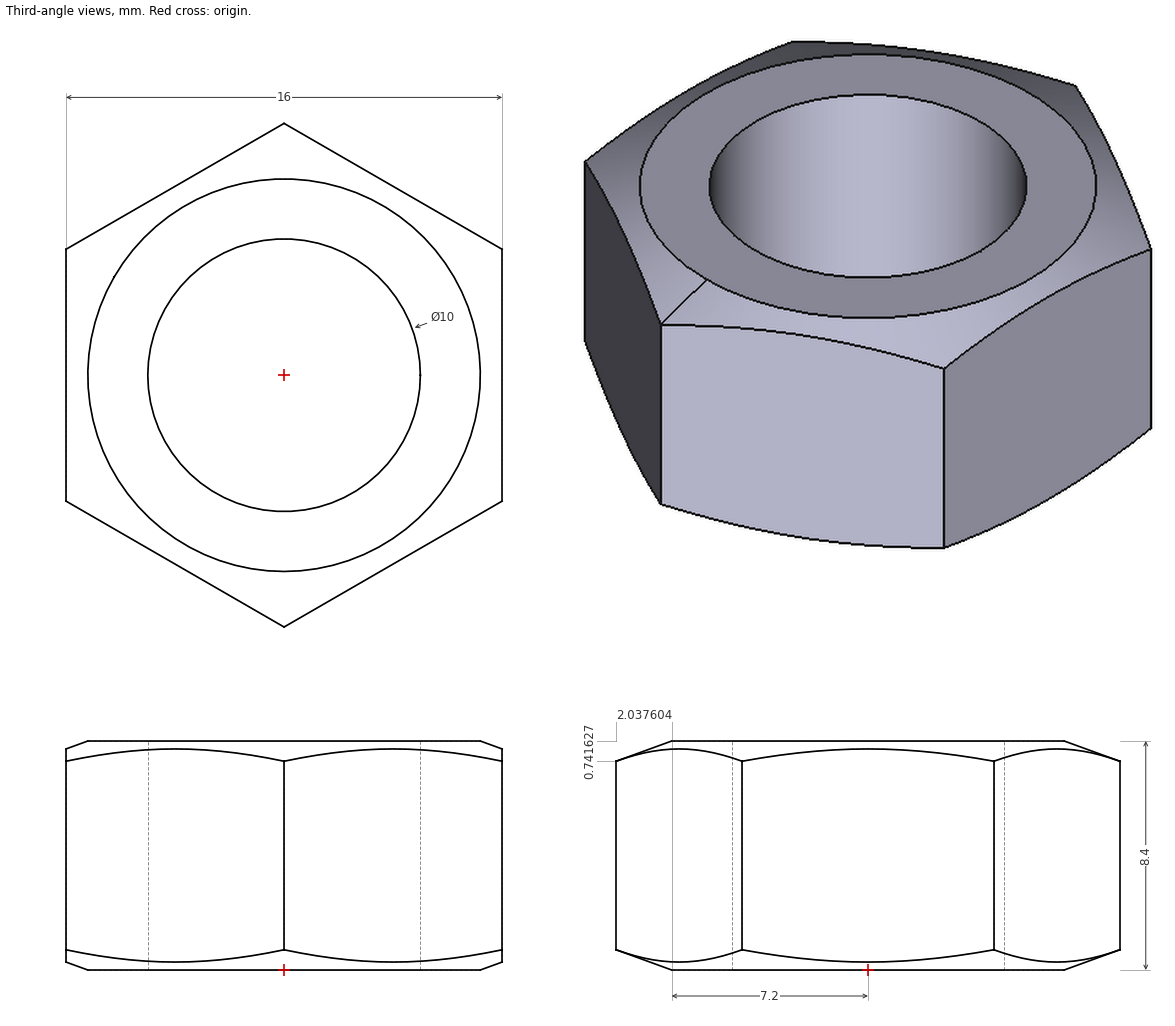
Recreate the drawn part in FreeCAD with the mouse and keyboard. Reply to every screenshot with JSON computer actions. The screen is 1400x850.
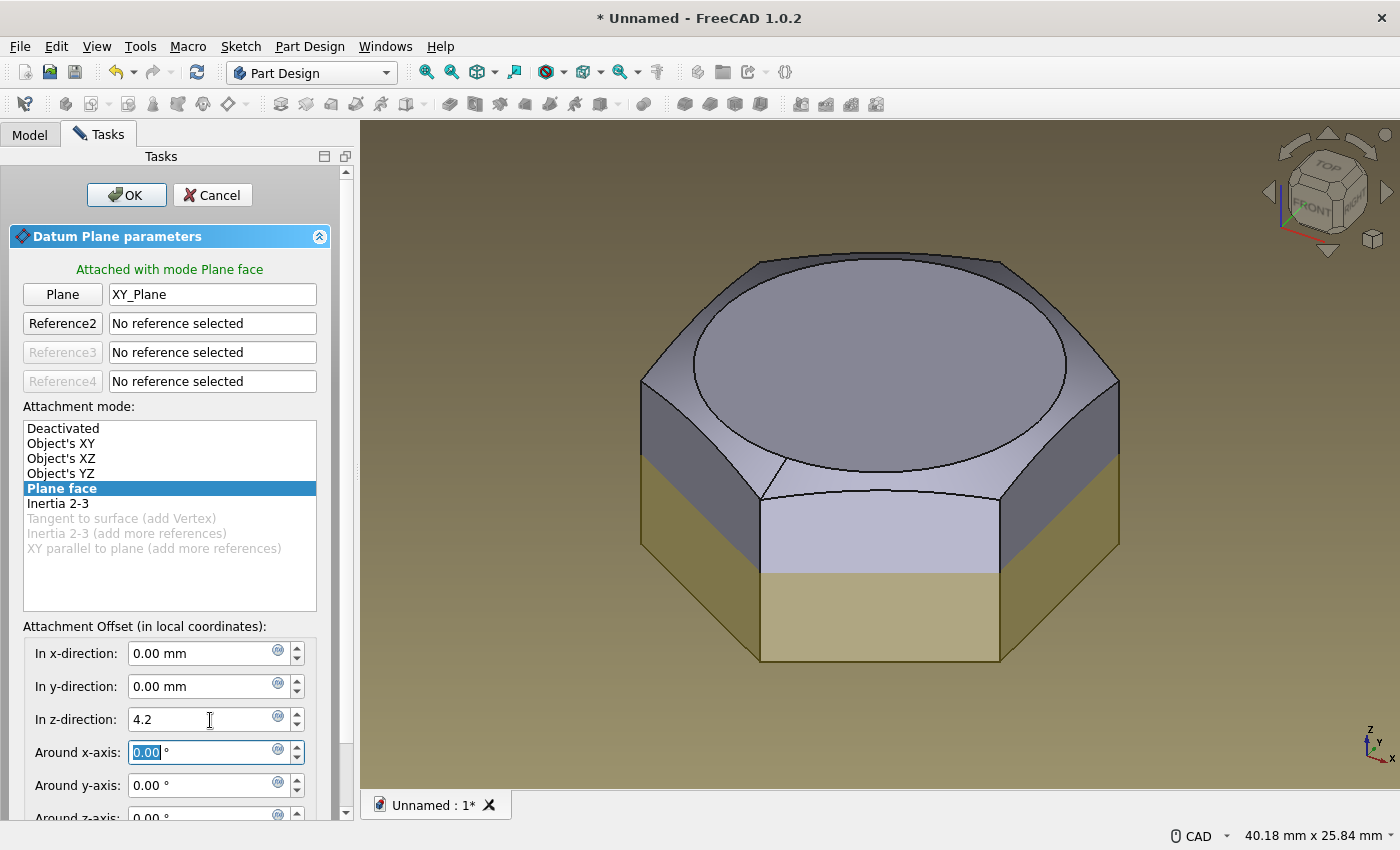
{"action": "left_click", "coordinate": [127, 195]}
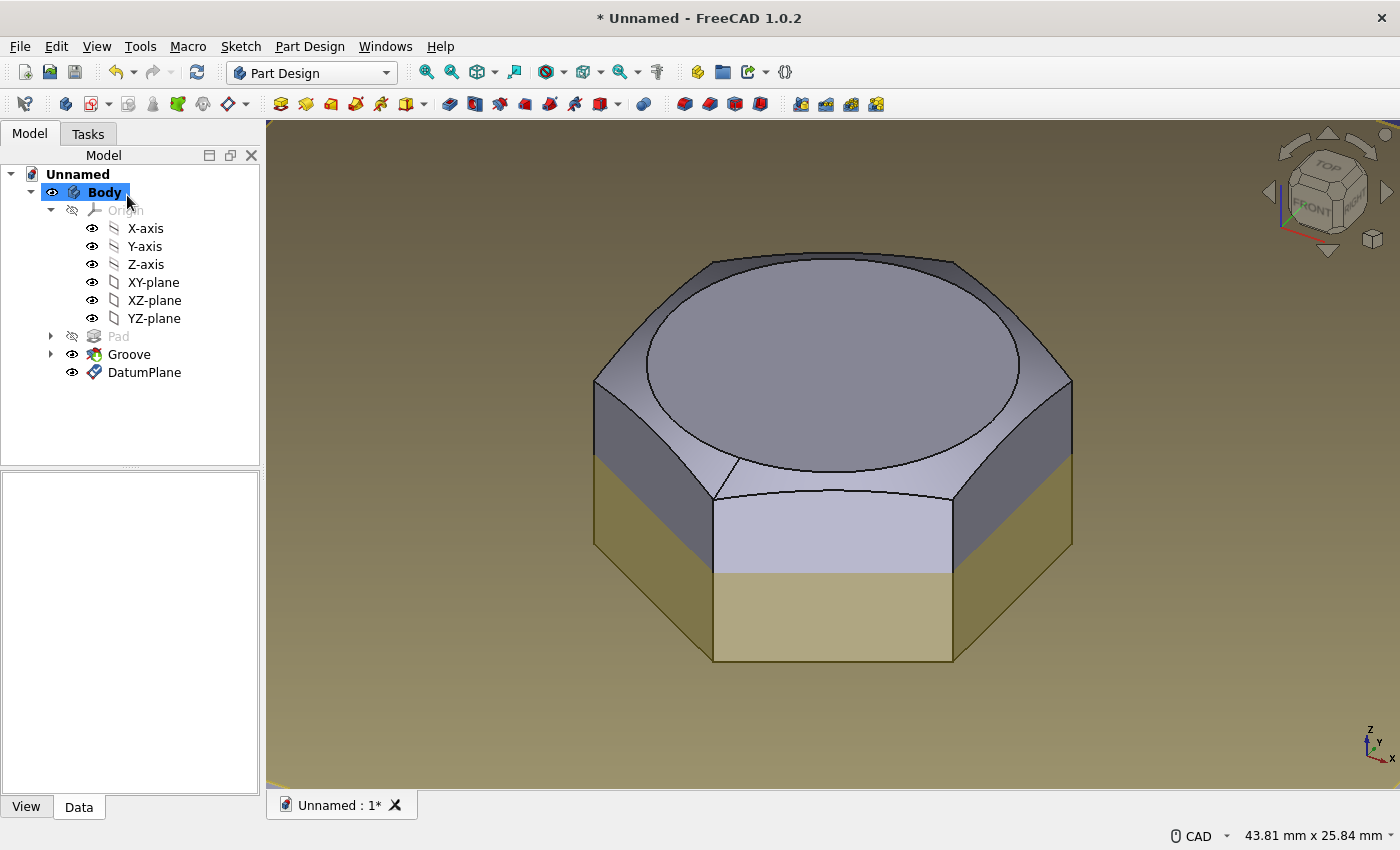
{"action": "left_click", "coordinate": [117, 354]}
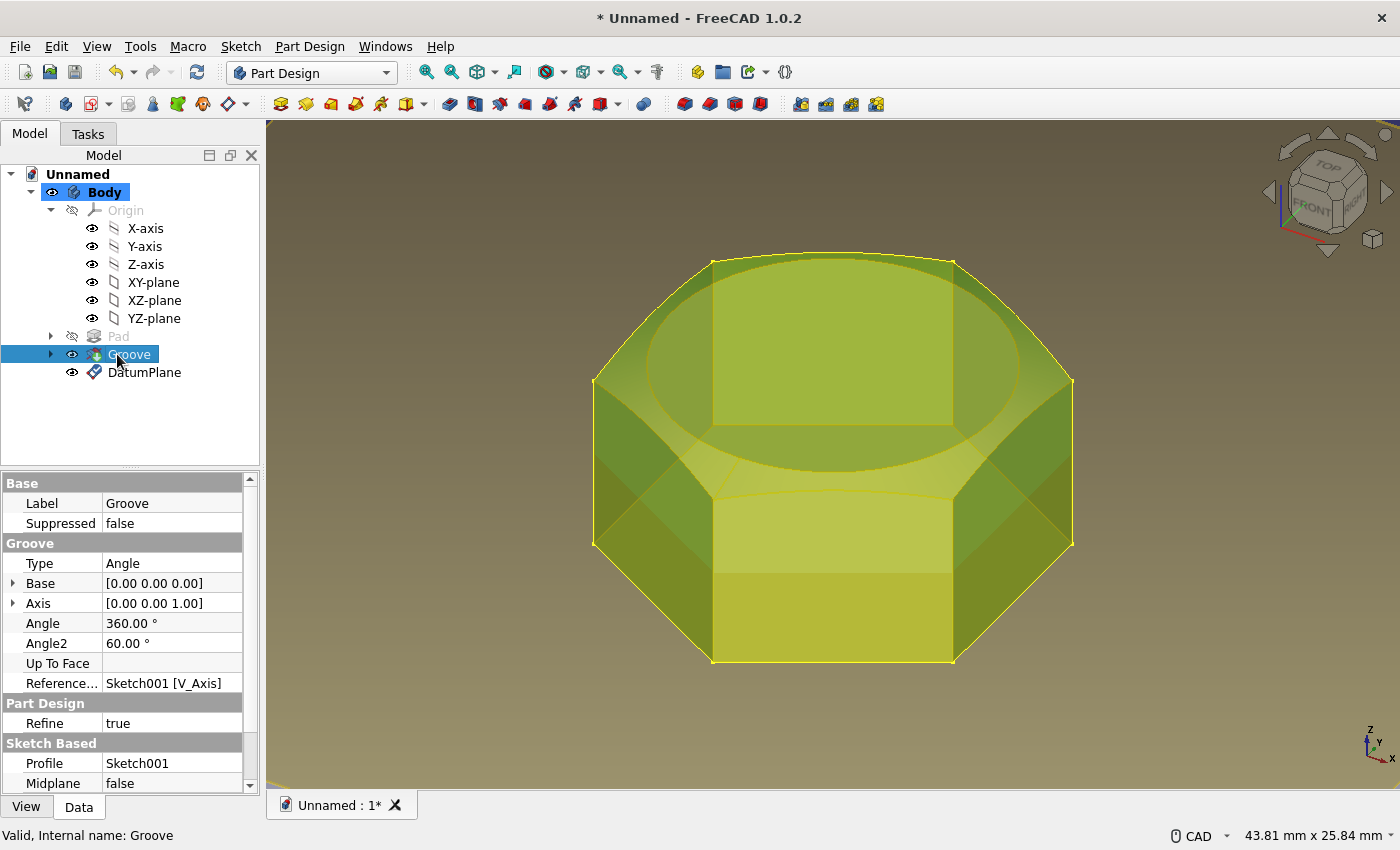
{"action": "left_click", "coordinate": [801, 104]}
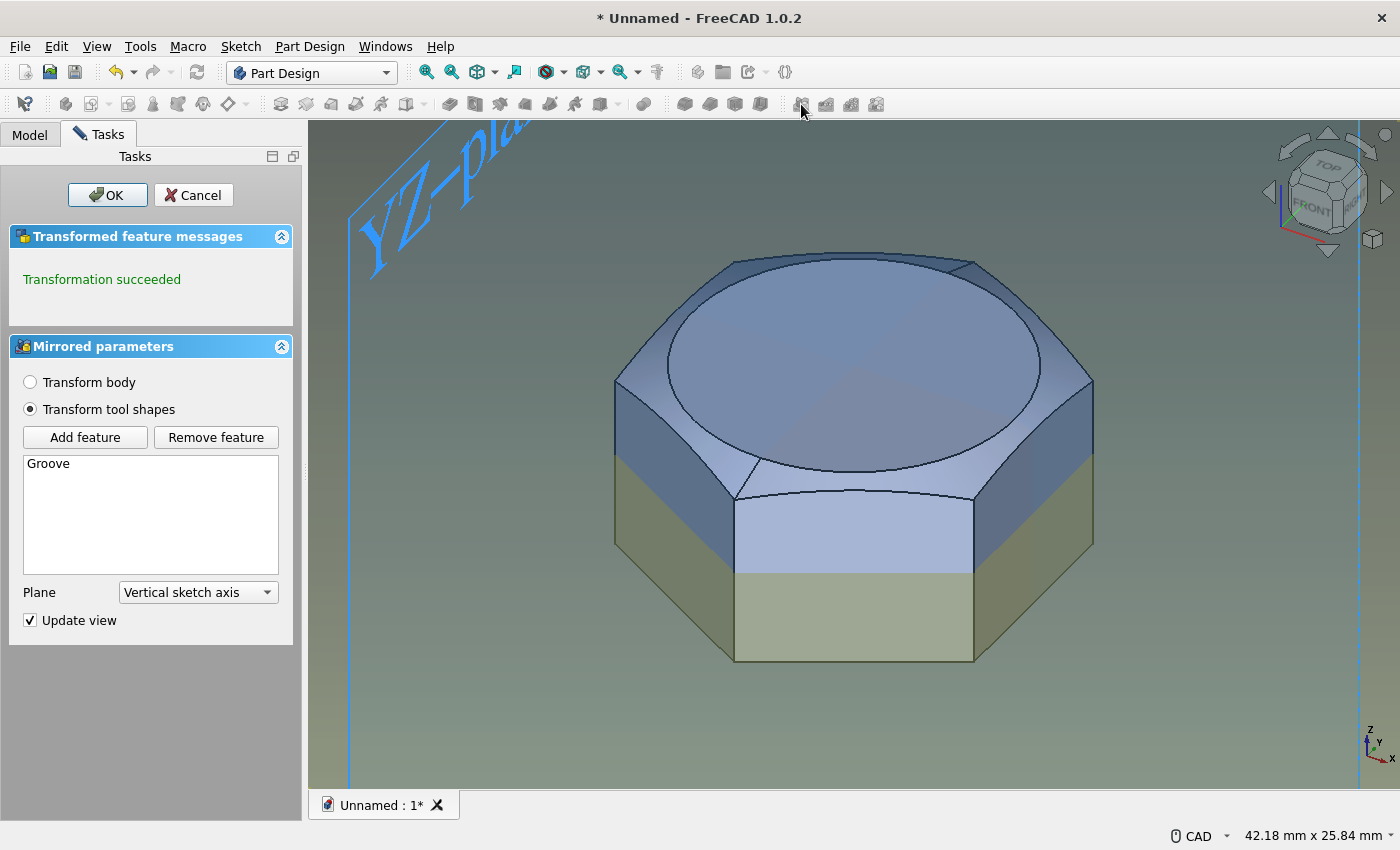
{"action": "left_click", "coordinate": [199, 592]}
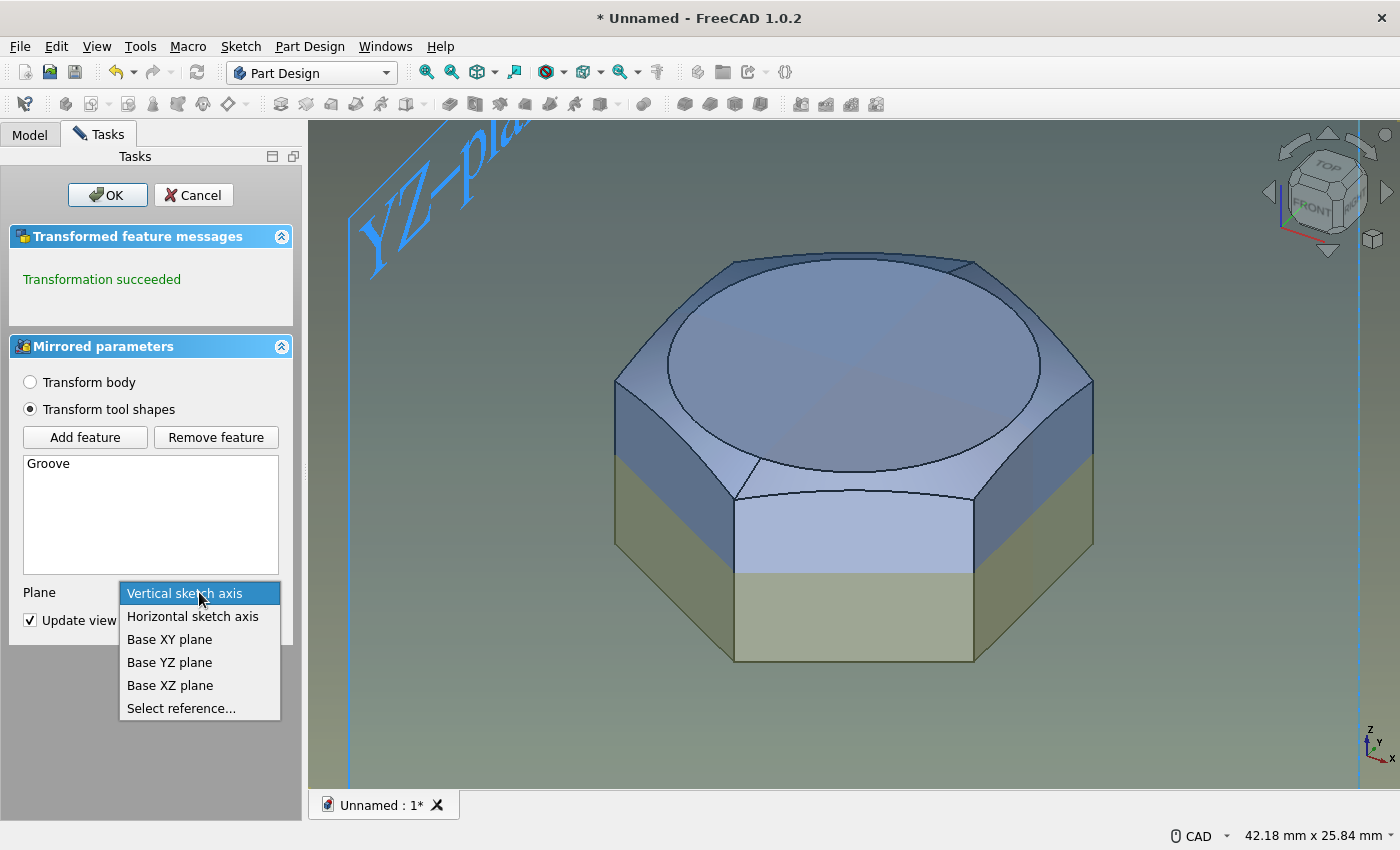
{"action": "left_click", "coordinate": [198, 708]}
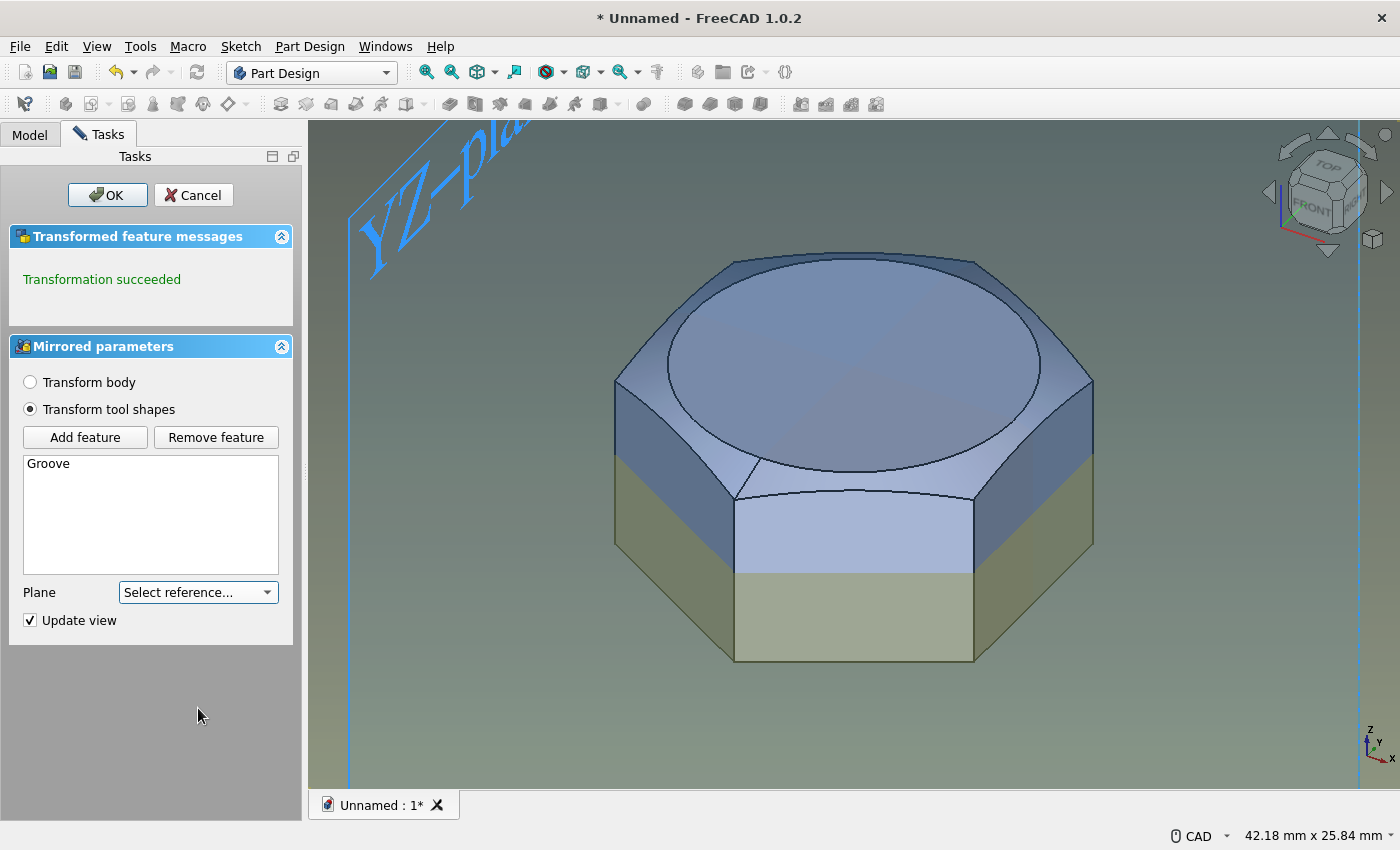
{"action": "left_click", "coordinate": [30, 134]}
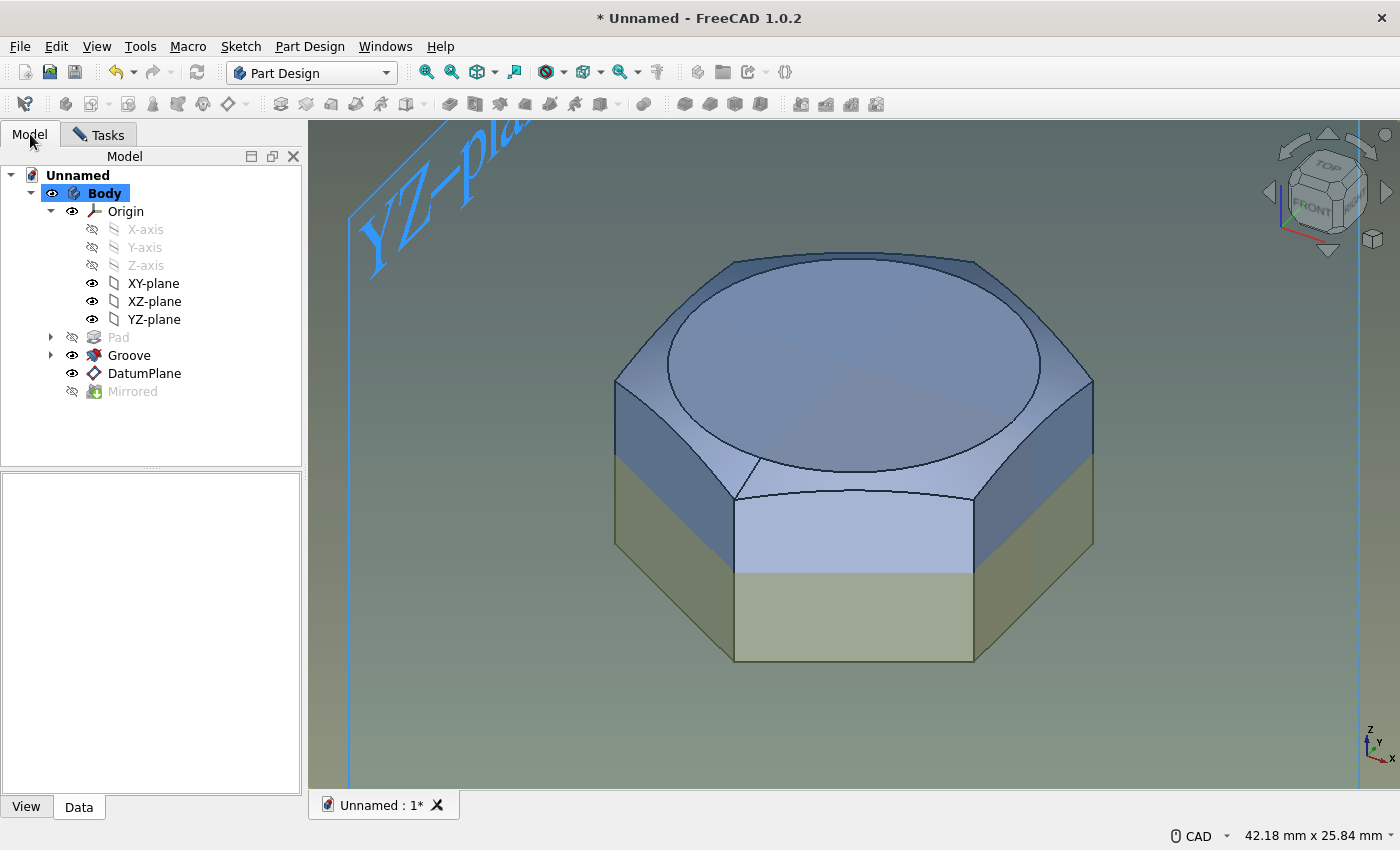
{"action": "left_click", "coordinate": [117, 373]}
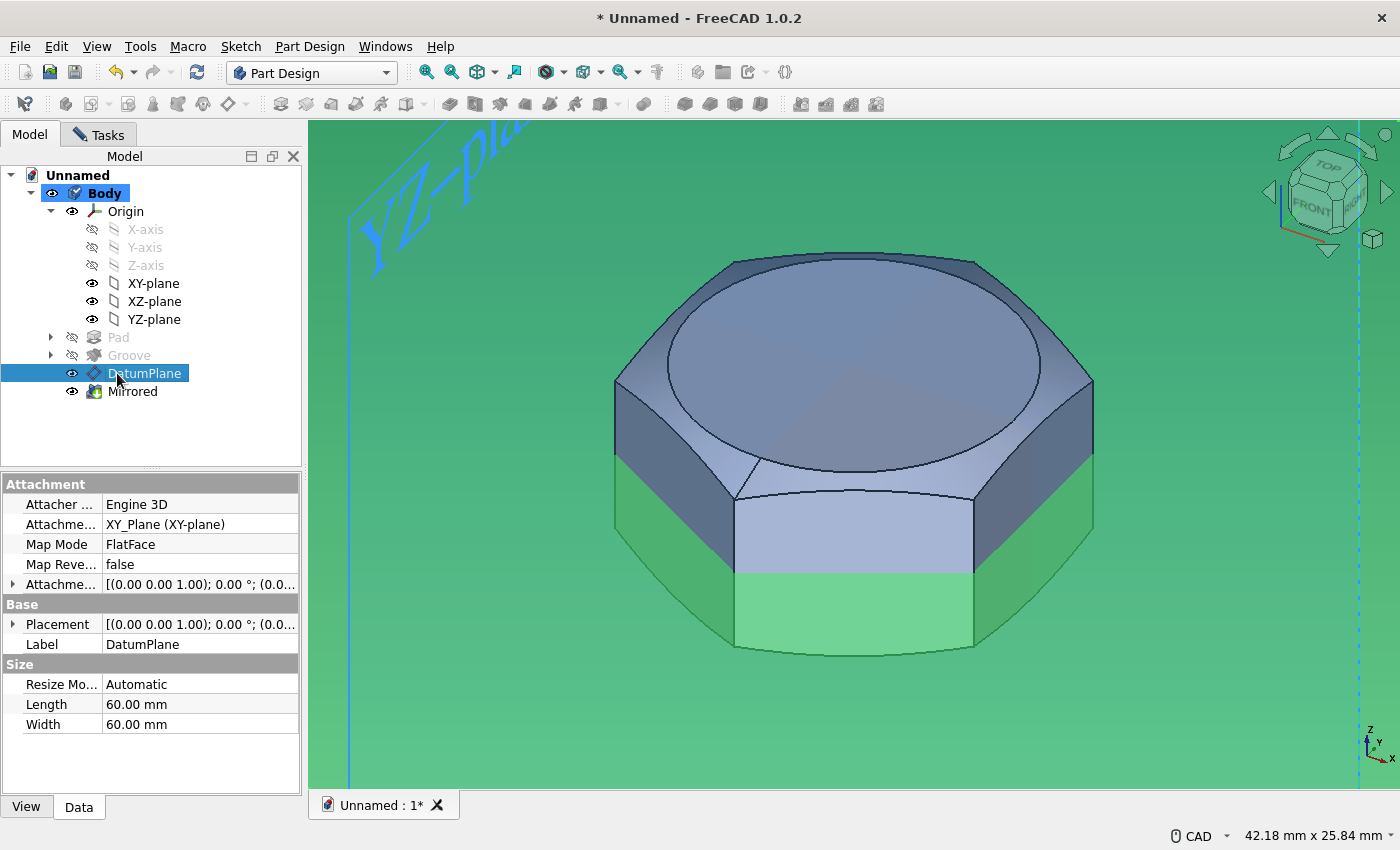
{"action": "left_click", "coordinate": [98, 134]}